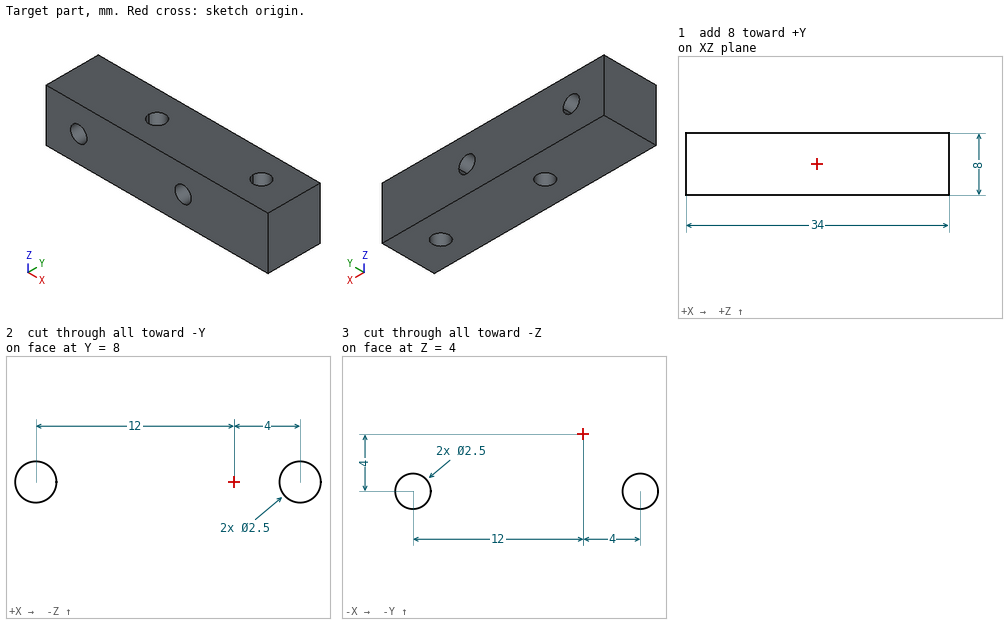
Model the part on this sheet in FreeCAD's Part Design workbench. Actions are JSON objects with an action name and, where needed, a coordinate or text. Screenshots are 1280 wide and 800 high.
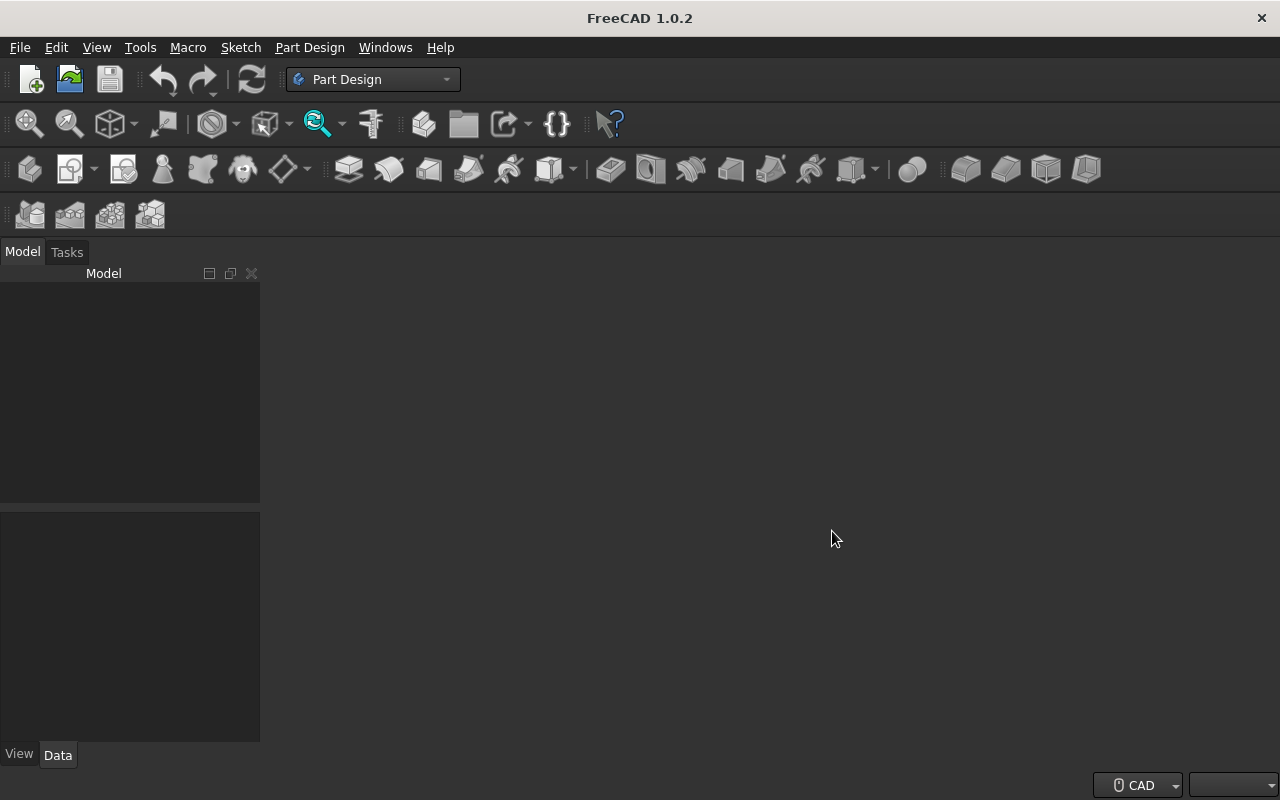
{"action": "left_click", "coordinate": [30, 80]}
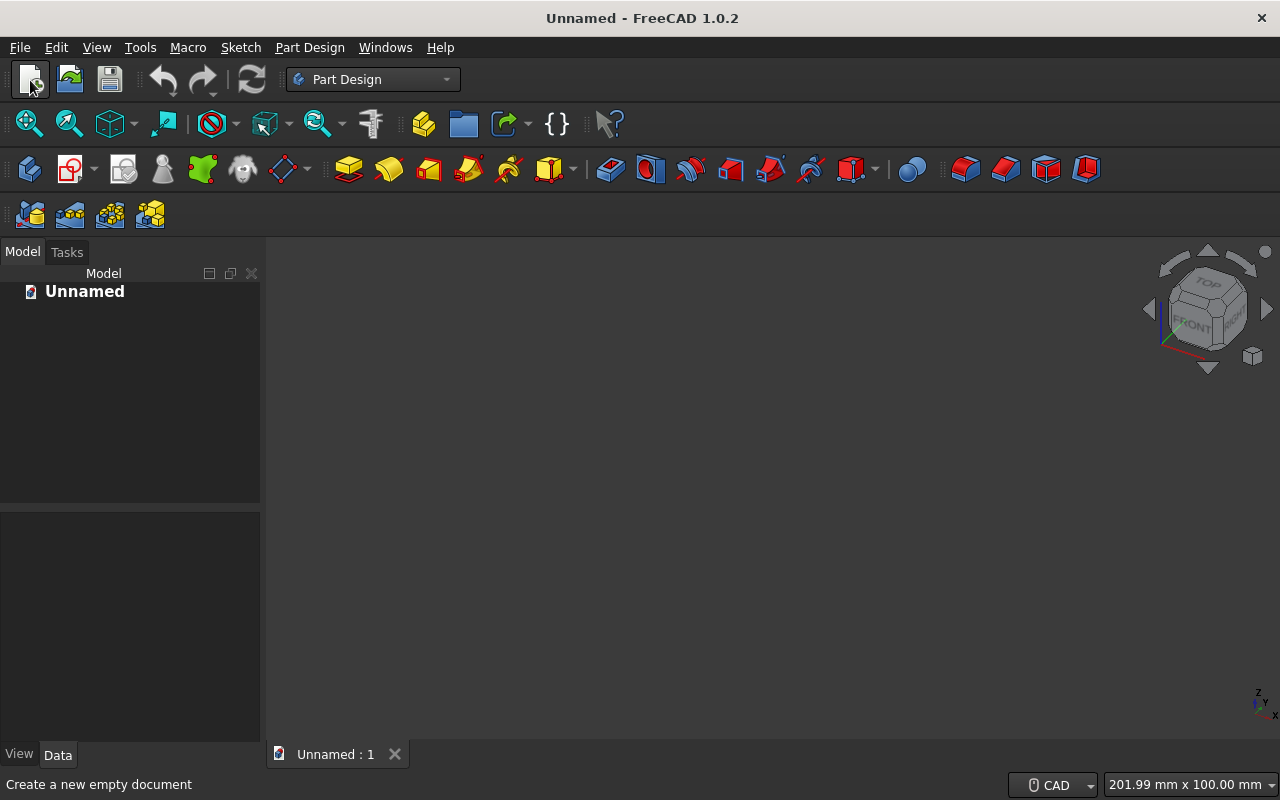
{"action": "left_click", "coordinate": [70, 170]}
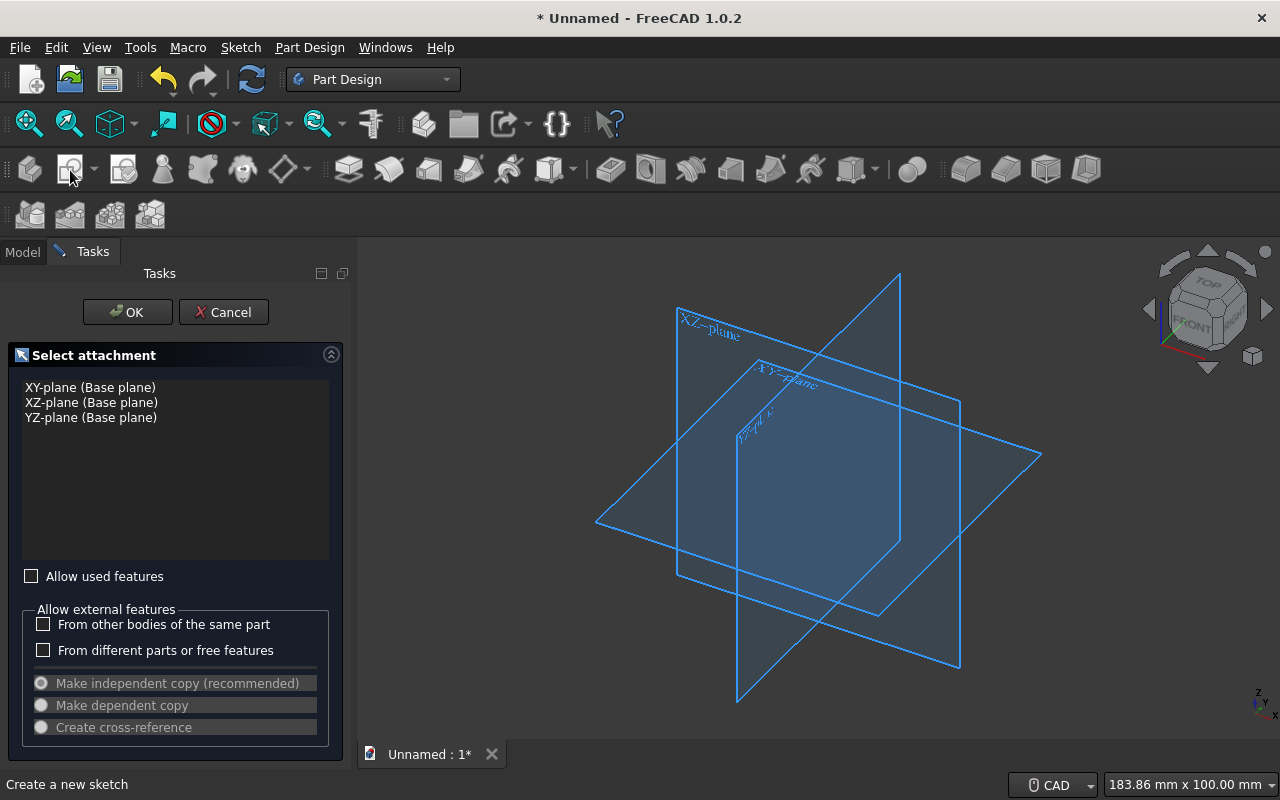
{"action": "left_click", "coordinate": [82, 402]}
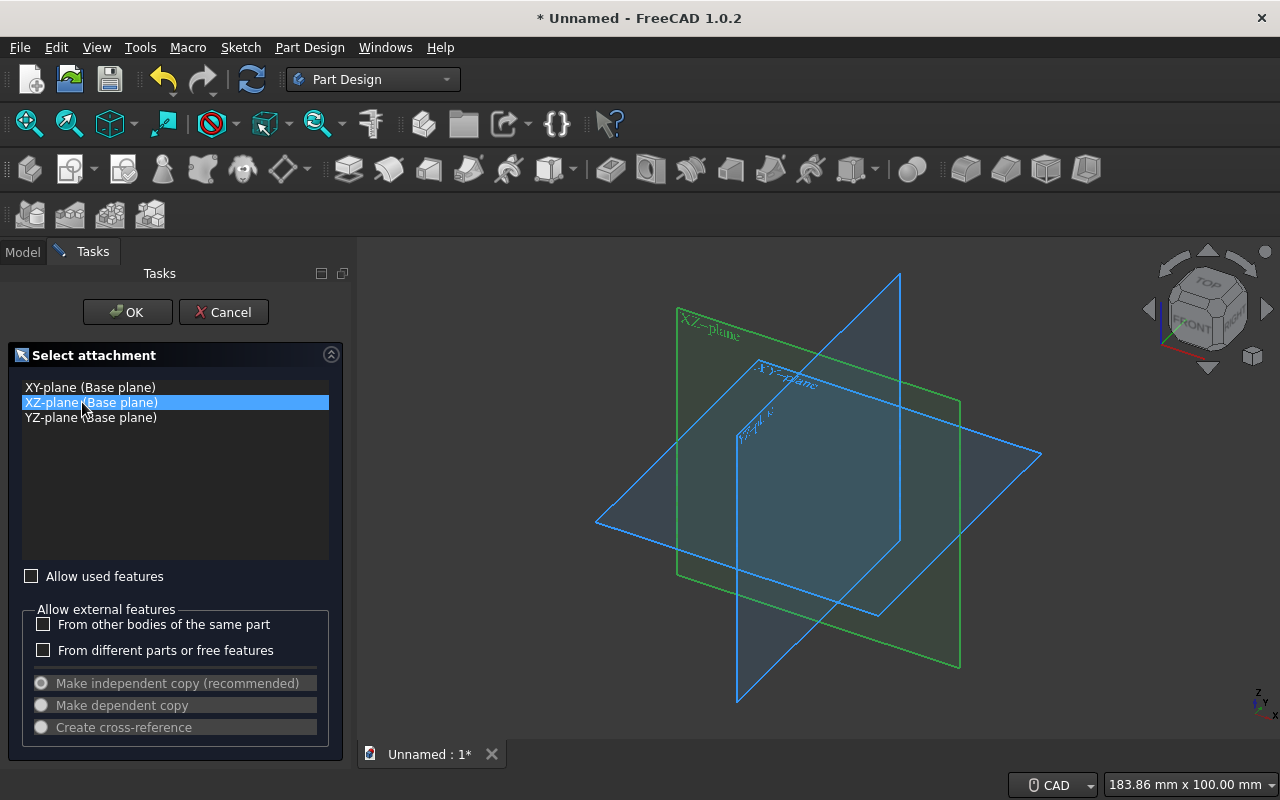
{"action": "left_click", "coordinate": [128, 312]}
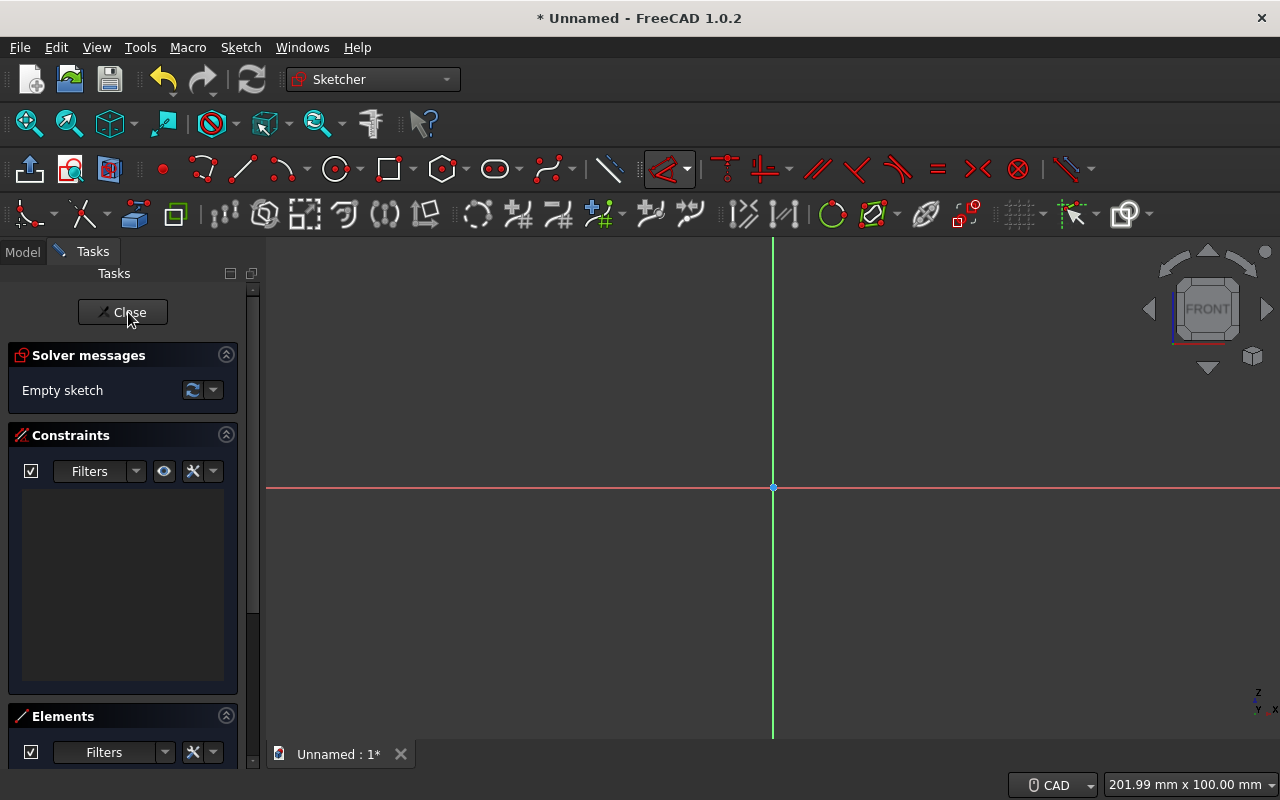
{"action": "scroll", "coordinate": [803, 488], "scroll_direction": "up", "scroll_amount": 6}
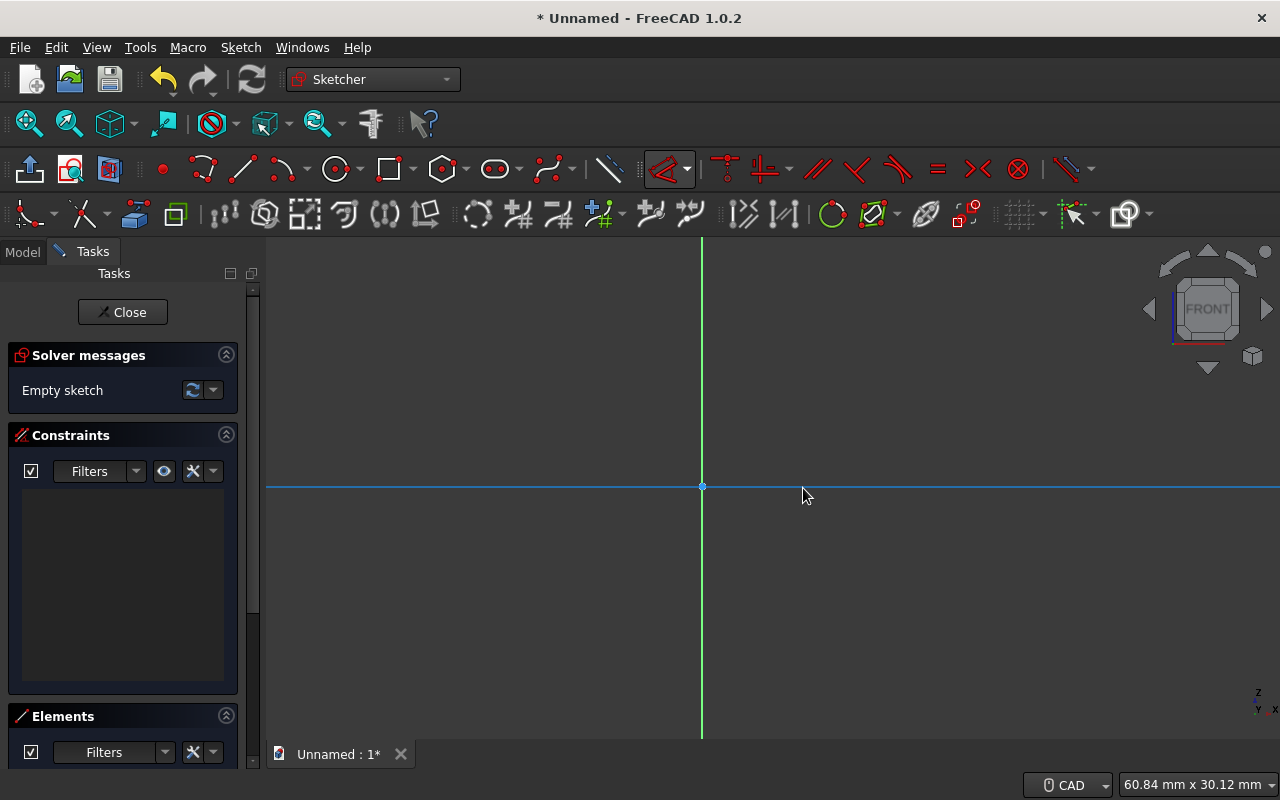
{"action": "left_click", "coordinate": [416, 170]}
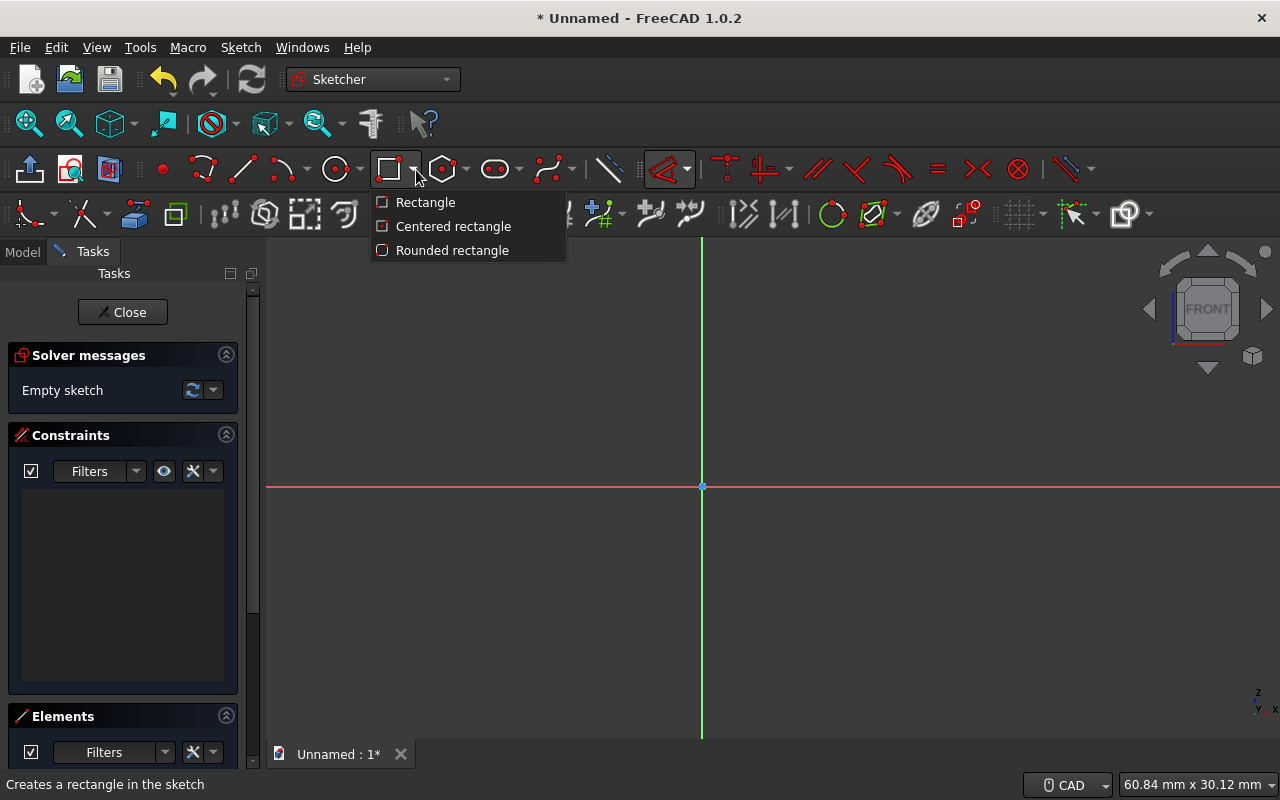
{"action": "left_click", "coordinate": [468, 226]}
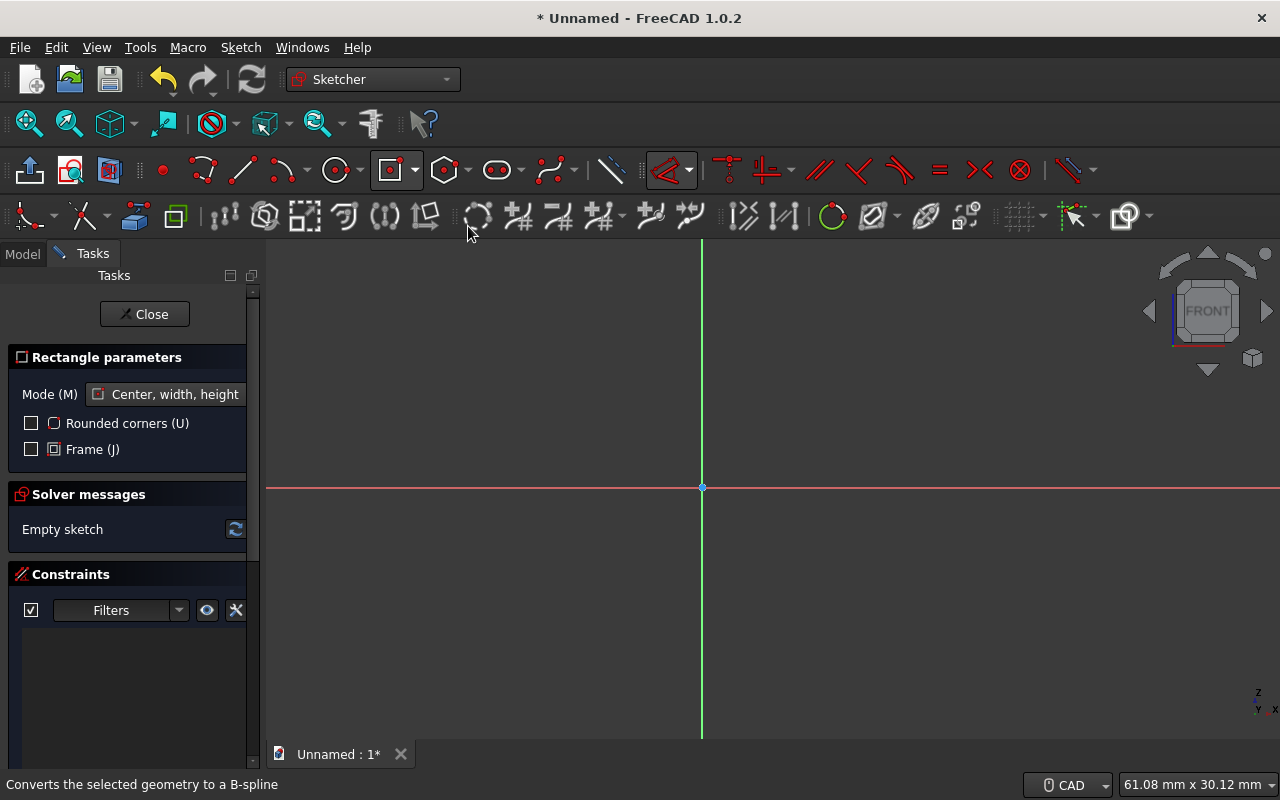
{"action": "left_click", "coordinate": [702, 488]}
{"action": "mouse_move", "coordinate": [985, 421]}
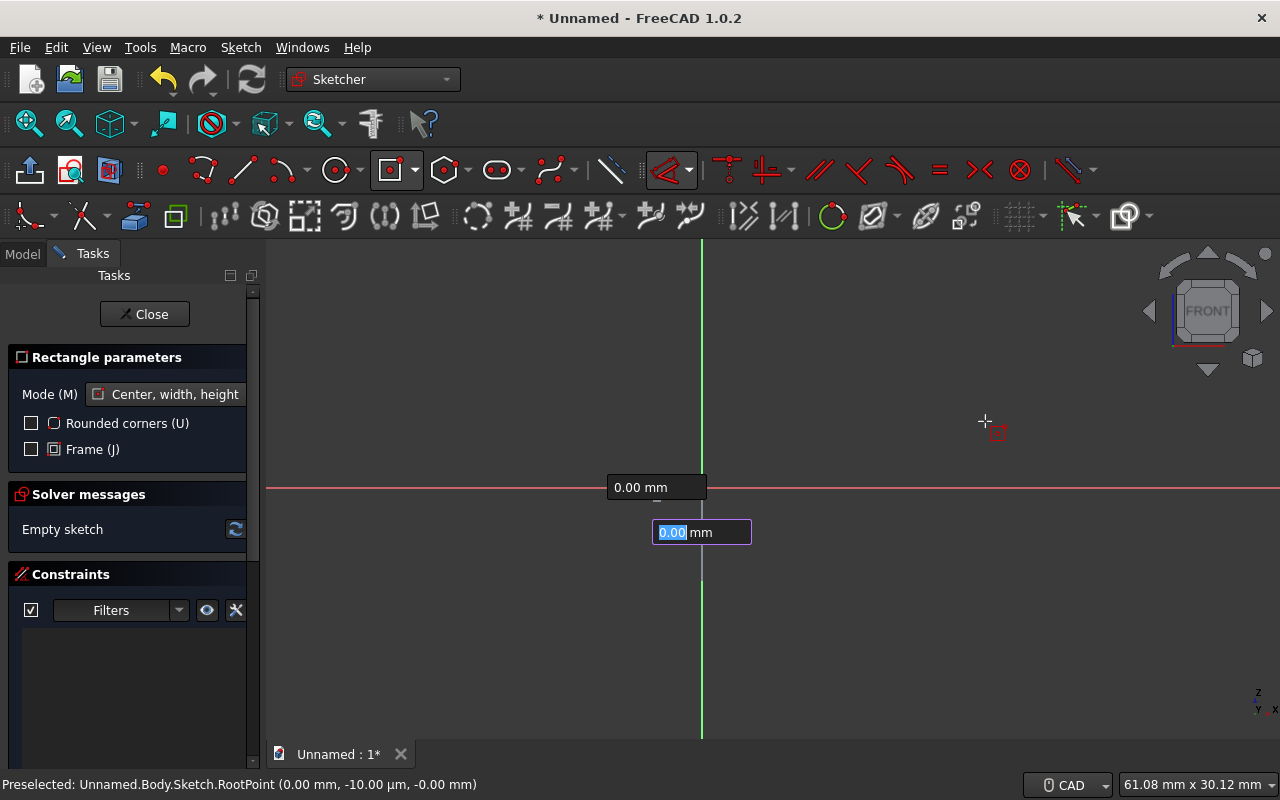
{"action": "type", "text": "34"}
{"action": "key", "text": "Tab"}
{"action": "type", "text": "8"}
{"action": "key", "text": "Return"}
{"action": "key", "text": "Escape"}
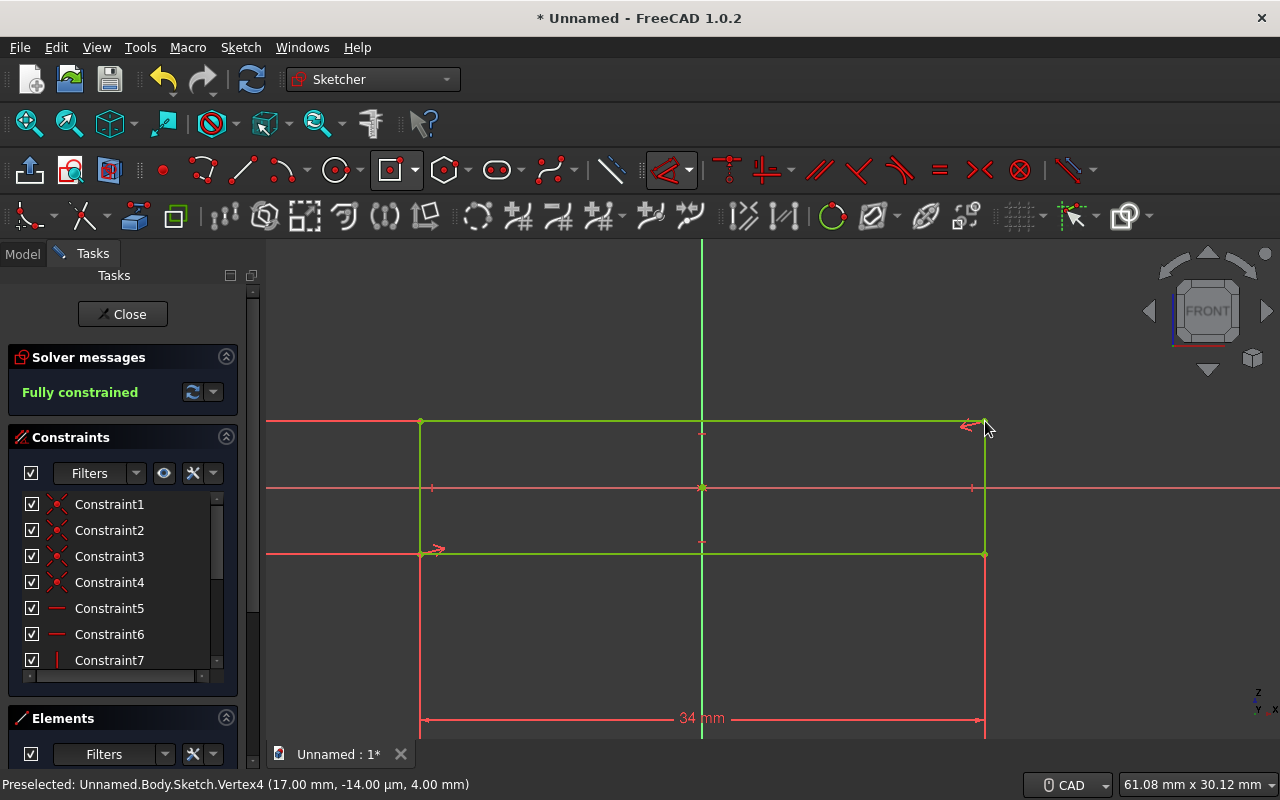
{"action": "left_click", "coordinate": [123, 314]}